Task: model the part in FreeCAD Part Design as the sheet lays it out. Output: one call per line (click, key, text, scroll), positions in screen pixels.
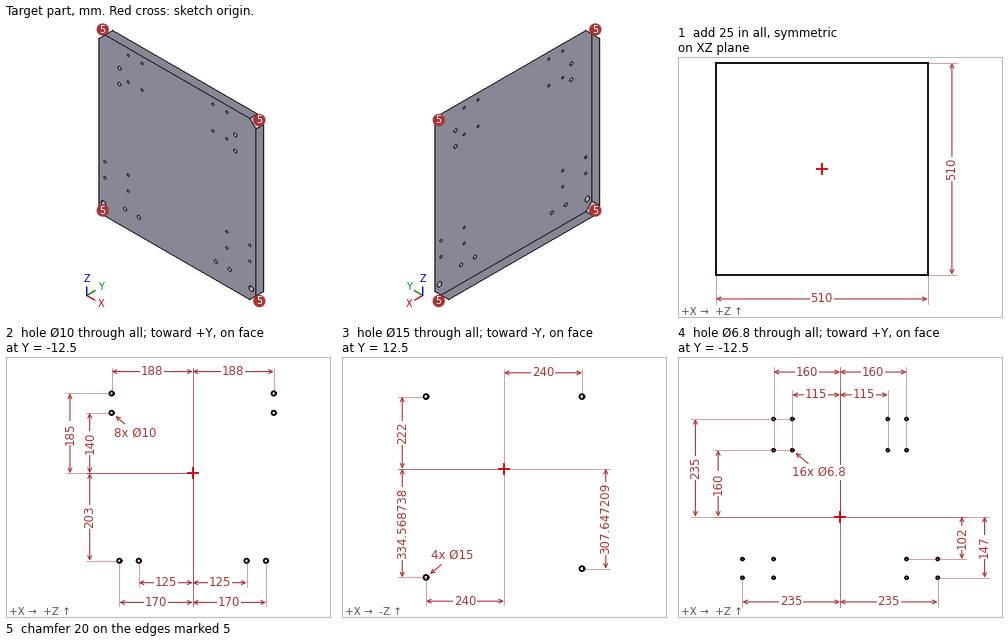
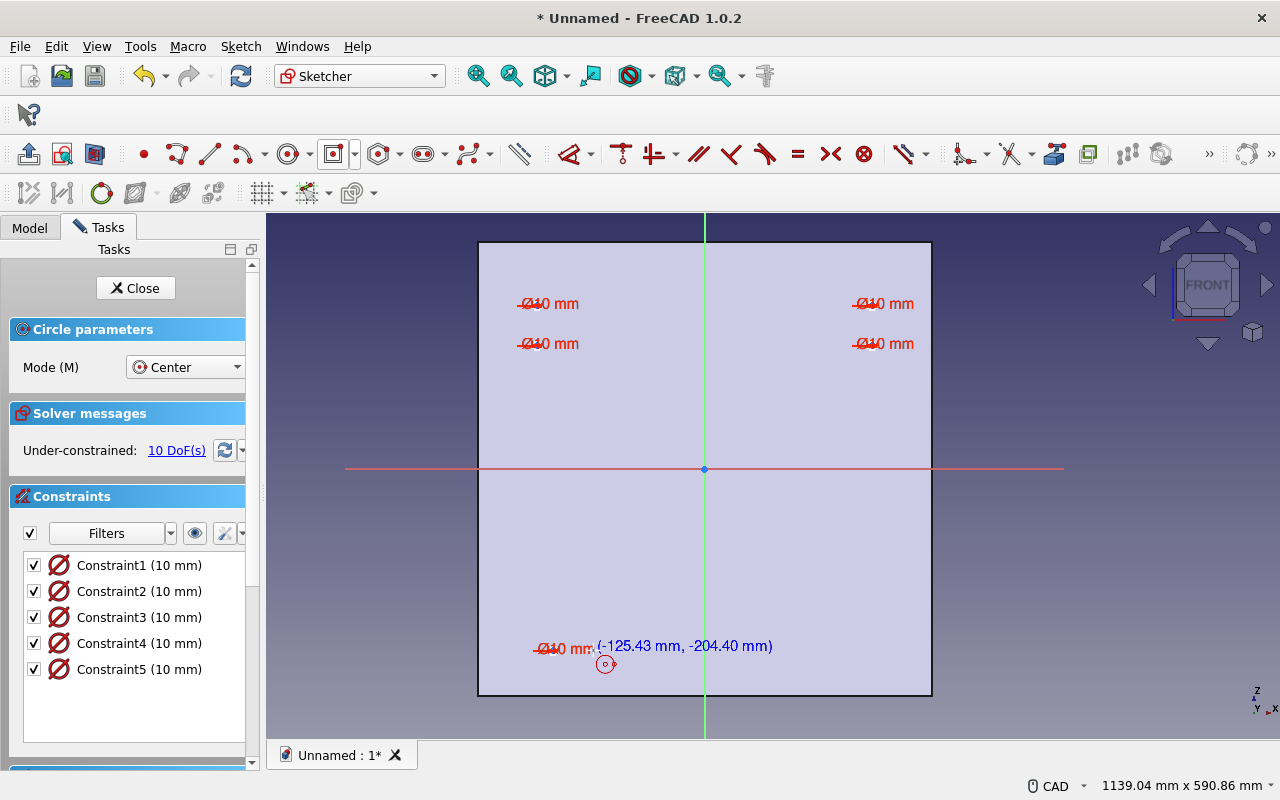
click(593, 650)
move(597, 647)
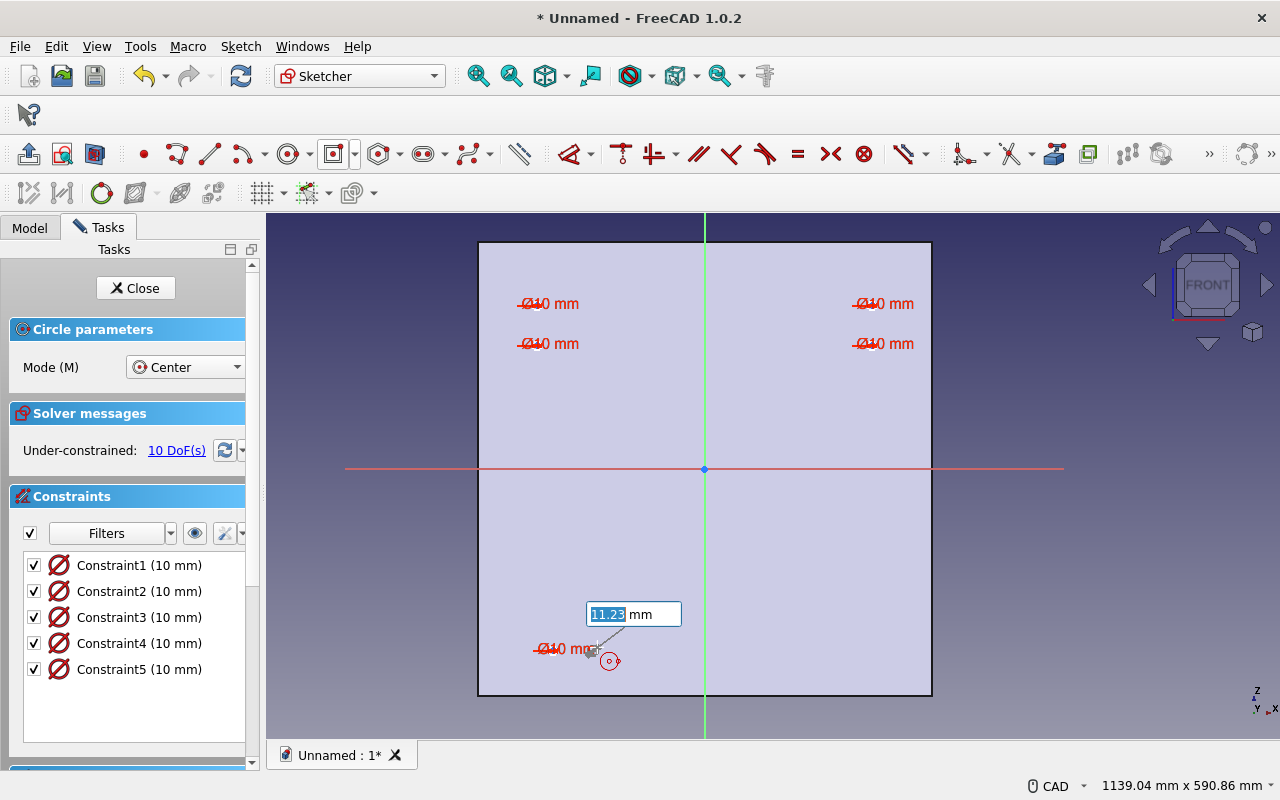
text(10)
key(Return)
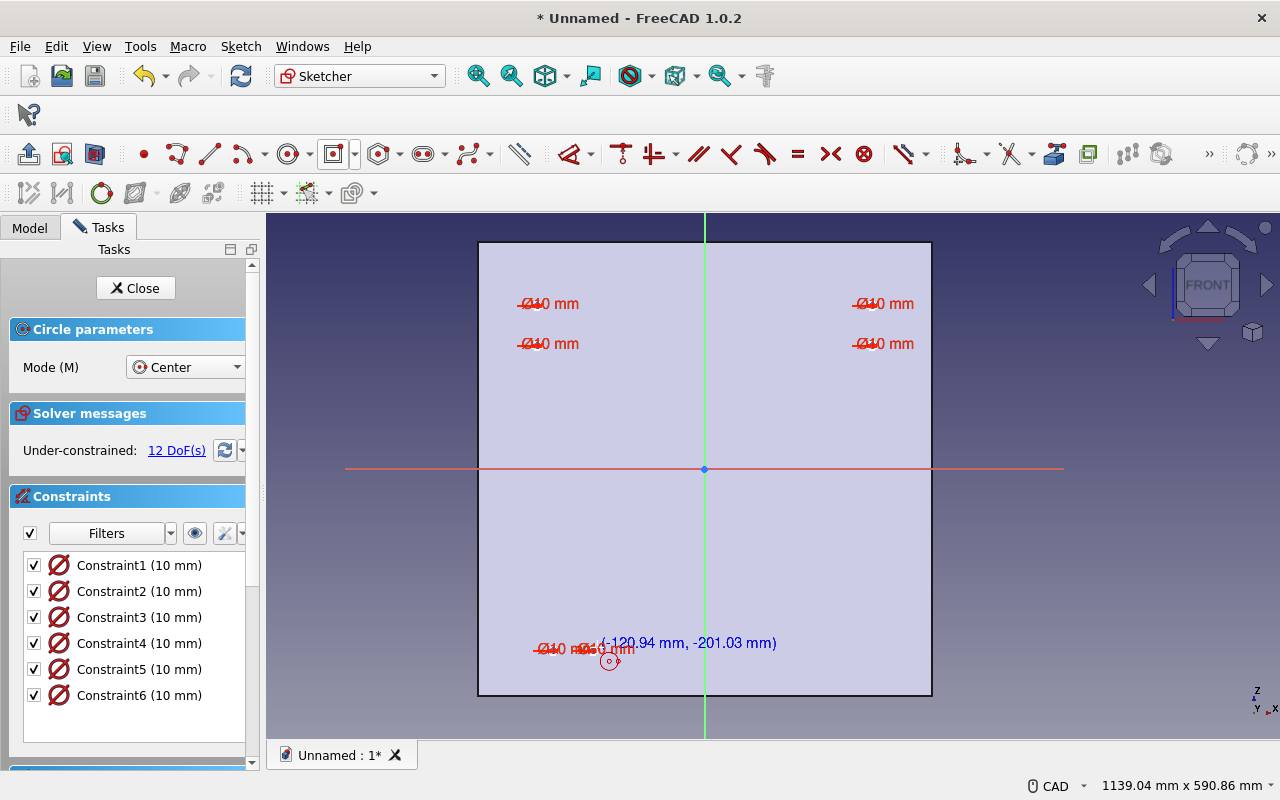
scroll(816, 650, up, 9)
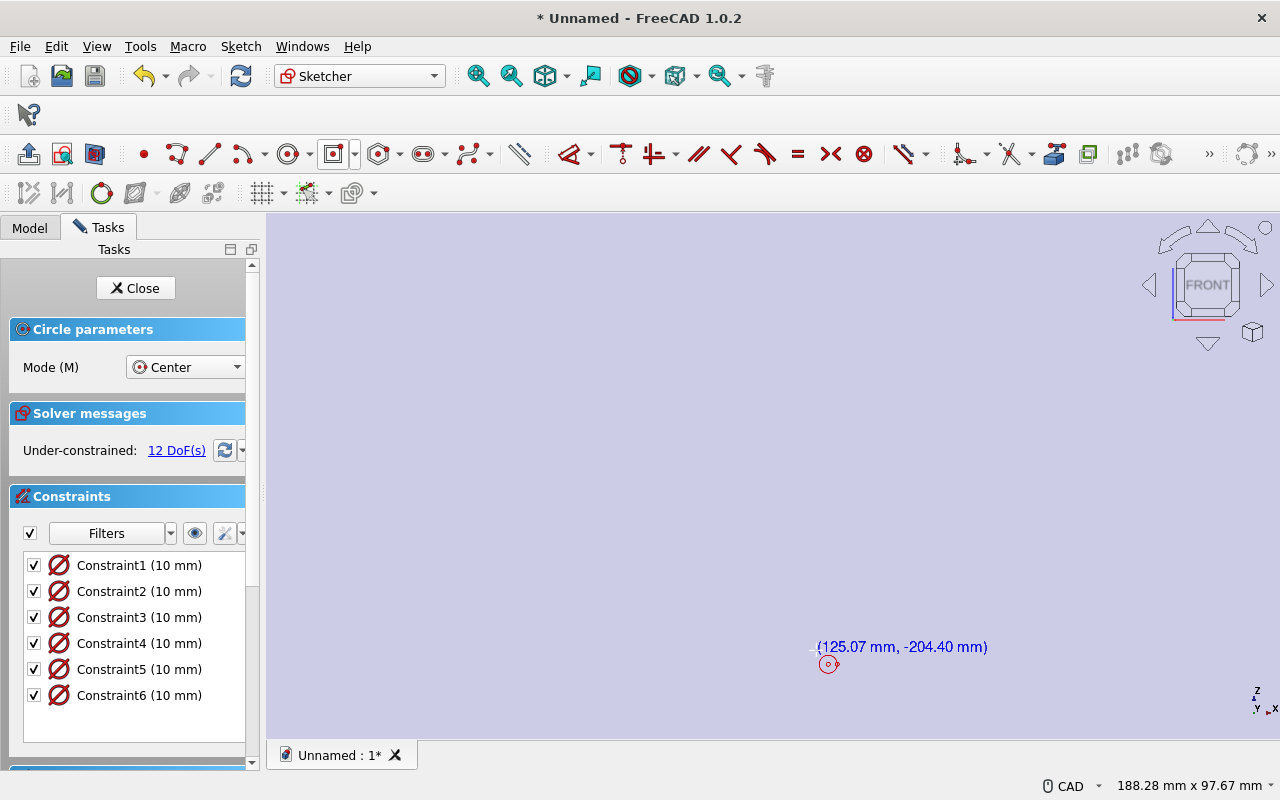
scroll(816, 650, down, 9)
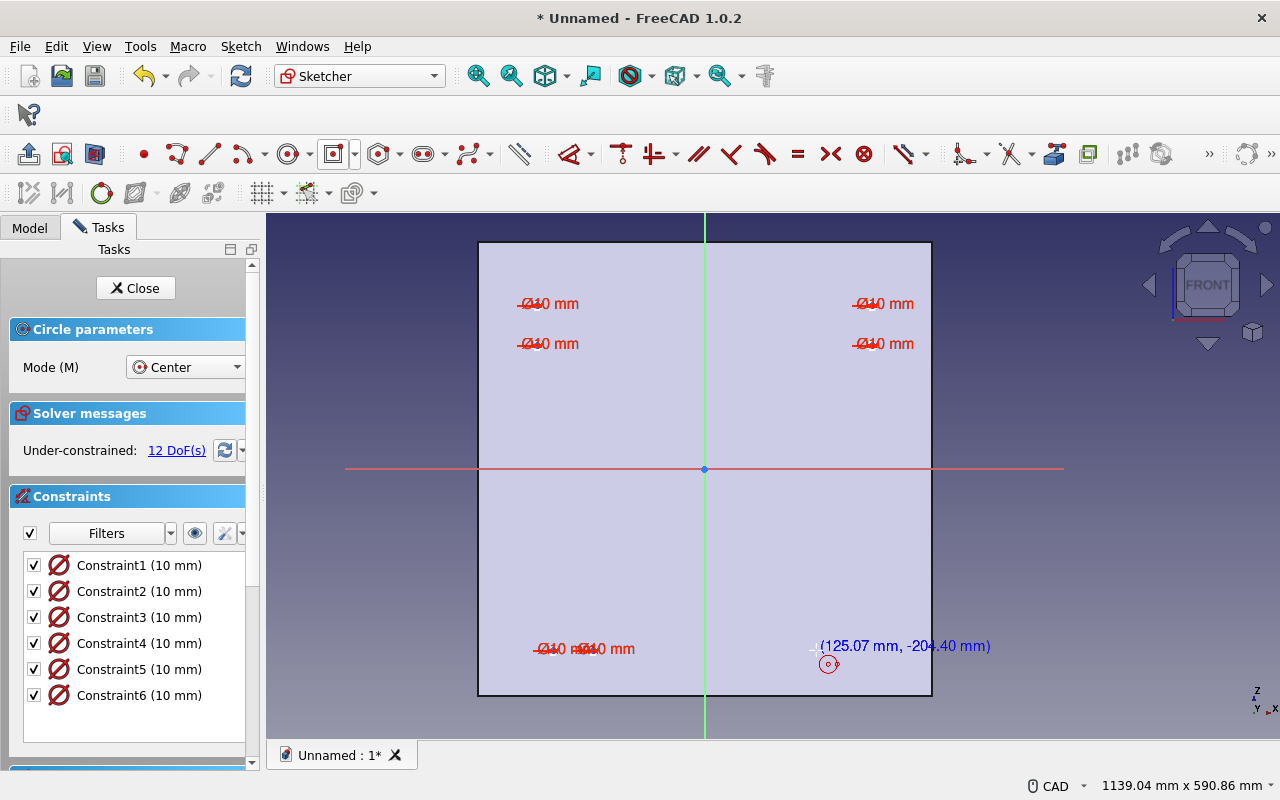
click(816, 650)
move(819, 647)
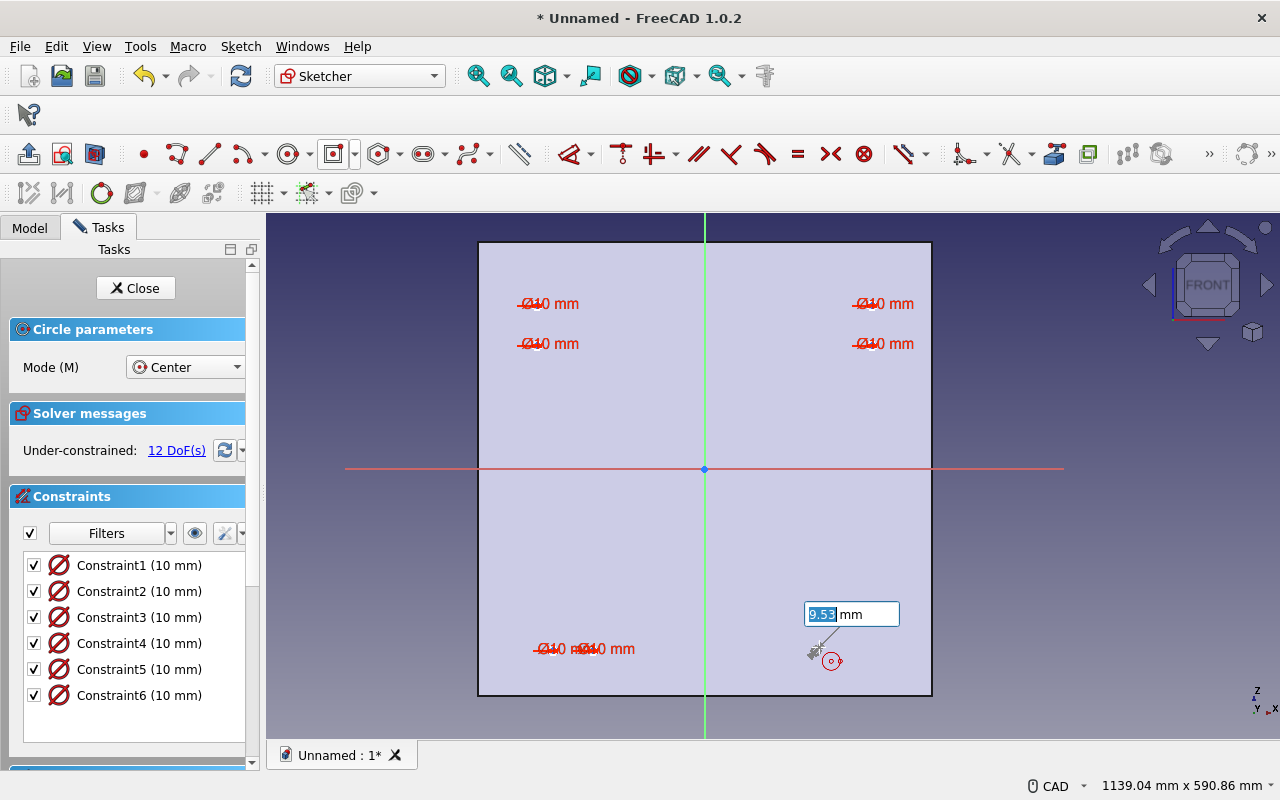
text(10)
key(Return)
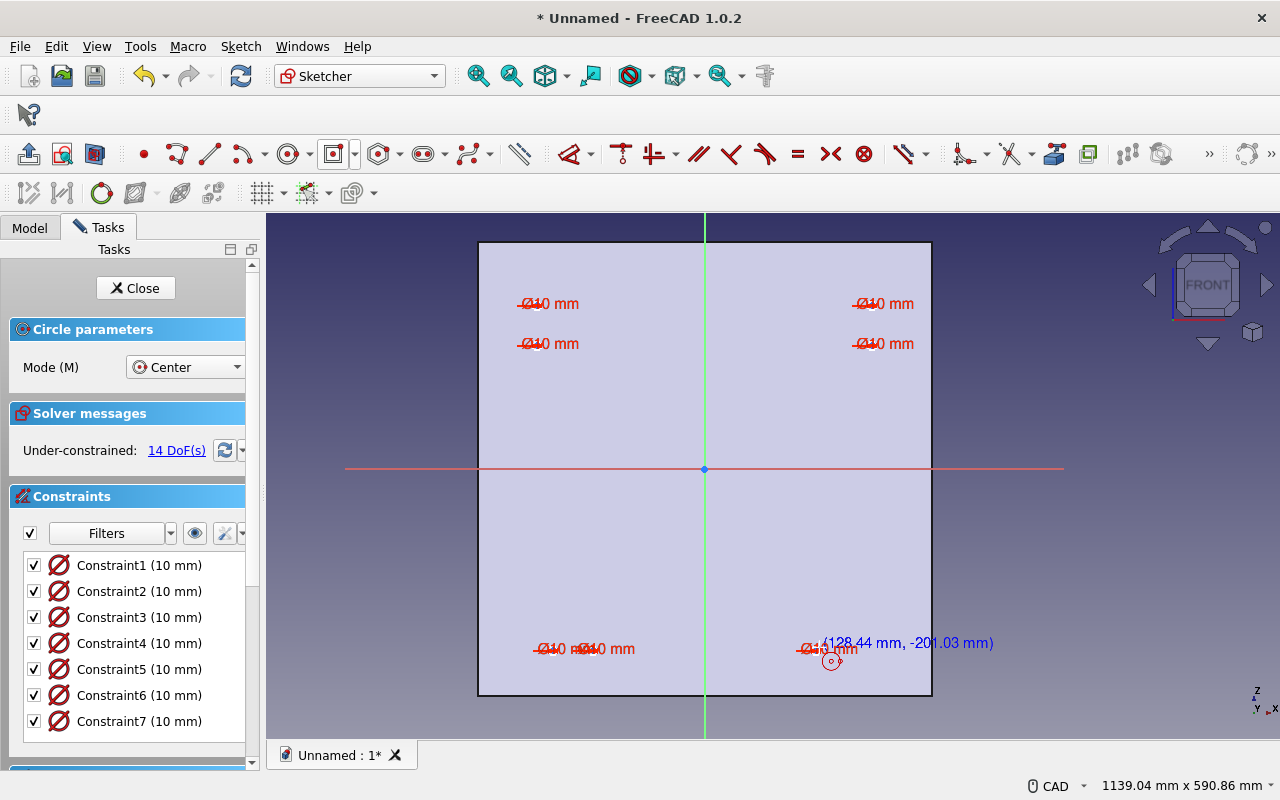
scroll(856, 650, up, 9)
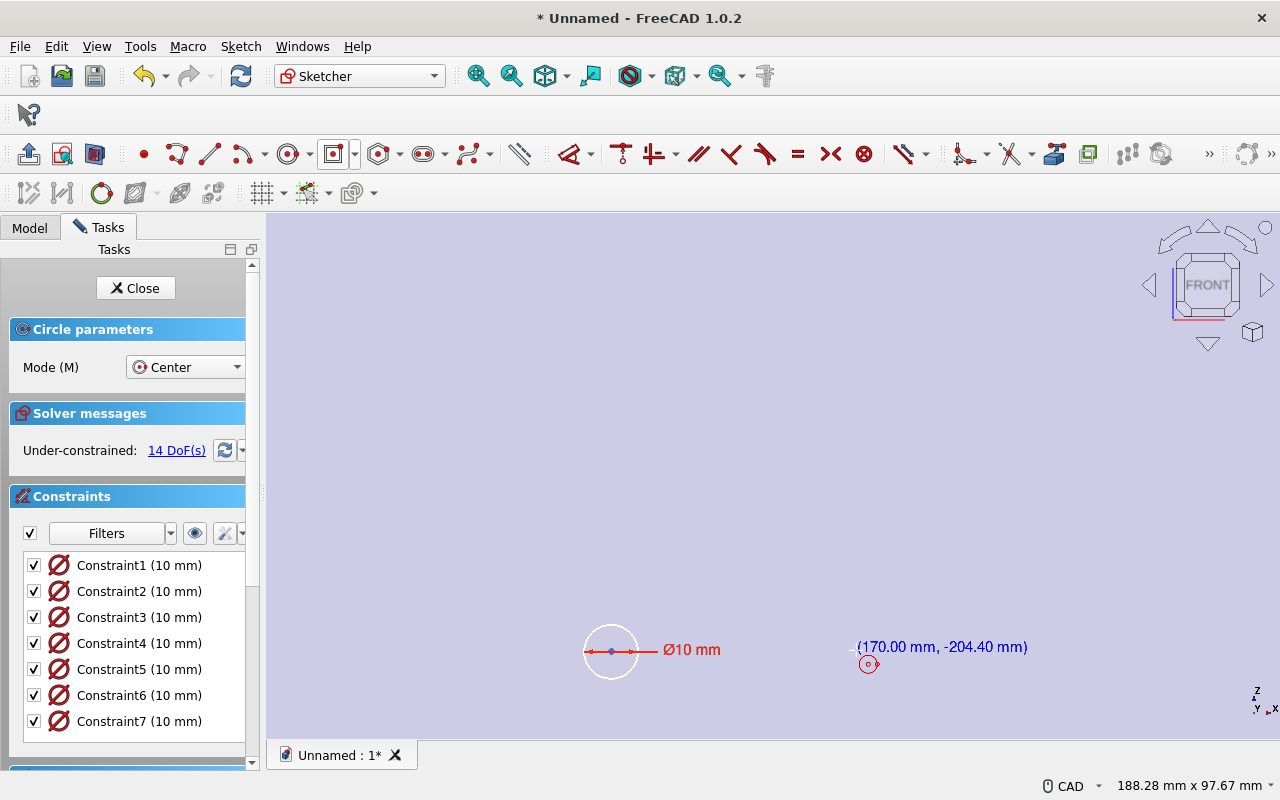
scroll(856, 650, down, 9)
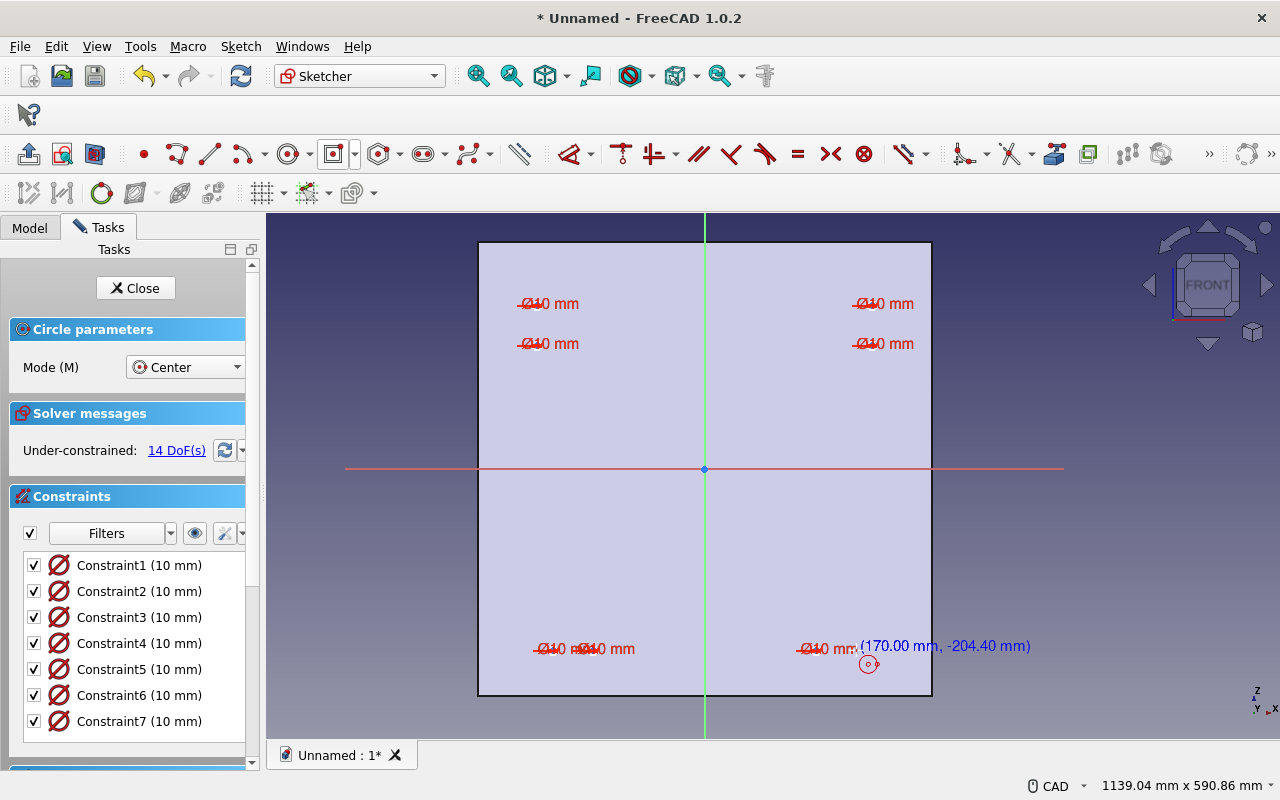
click(856, 650)
move(859, 647)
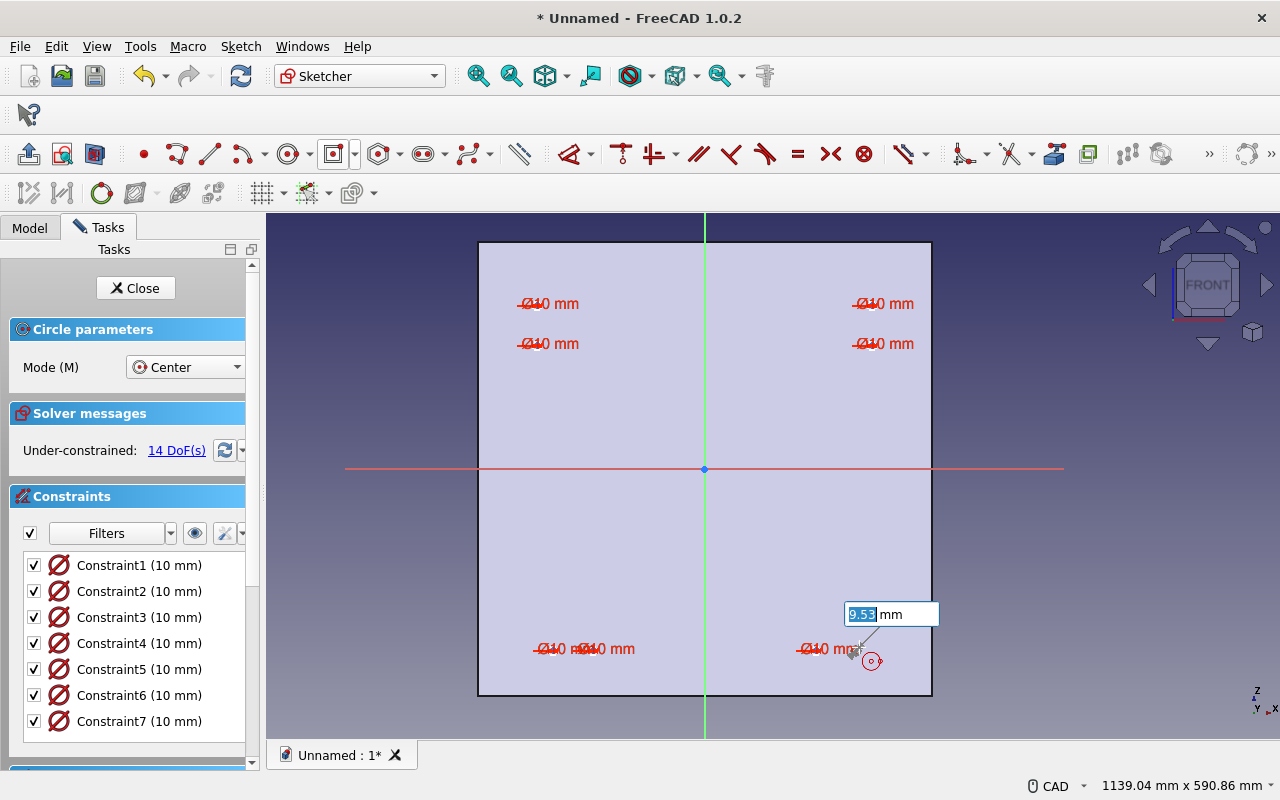
text(10)
key(Return)
key(Escape)